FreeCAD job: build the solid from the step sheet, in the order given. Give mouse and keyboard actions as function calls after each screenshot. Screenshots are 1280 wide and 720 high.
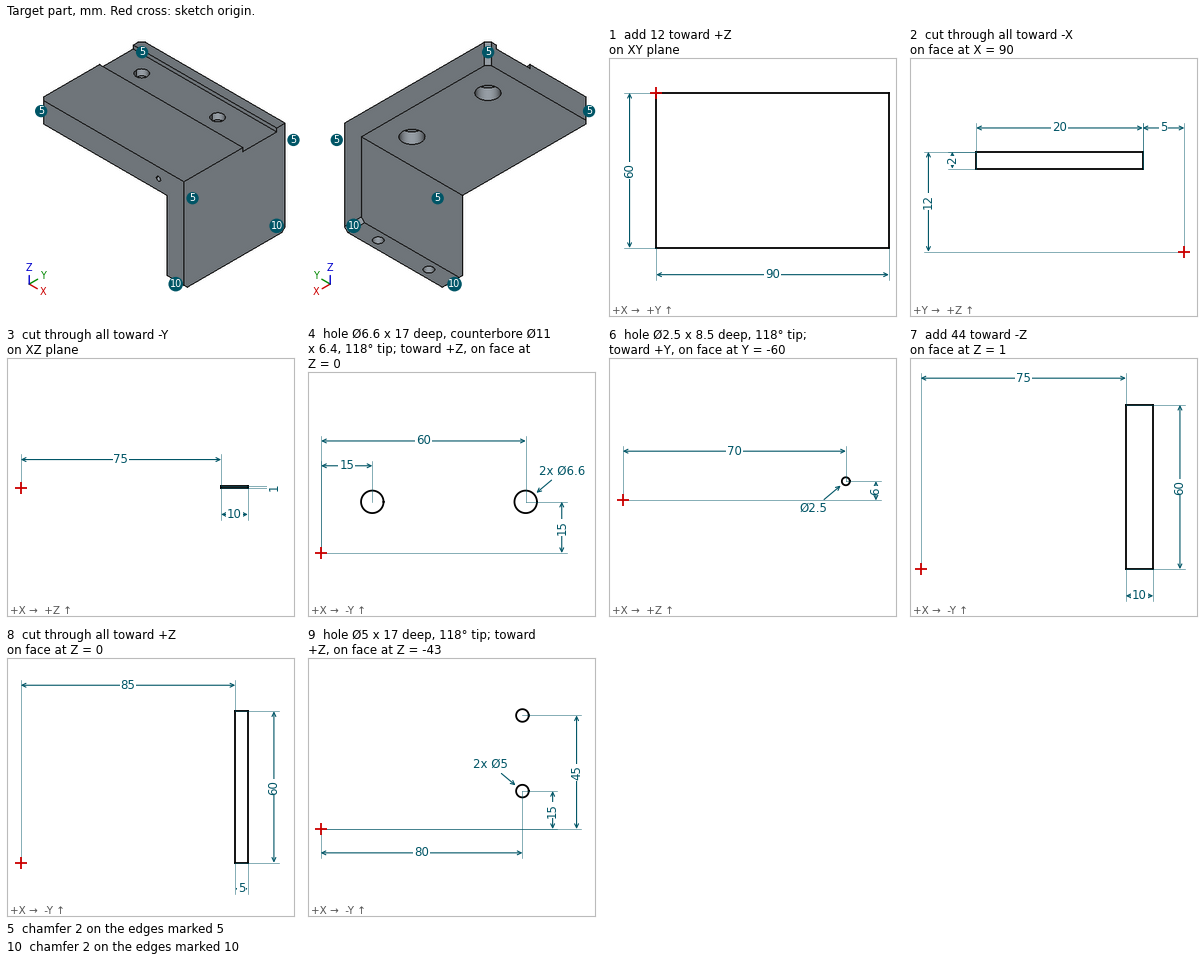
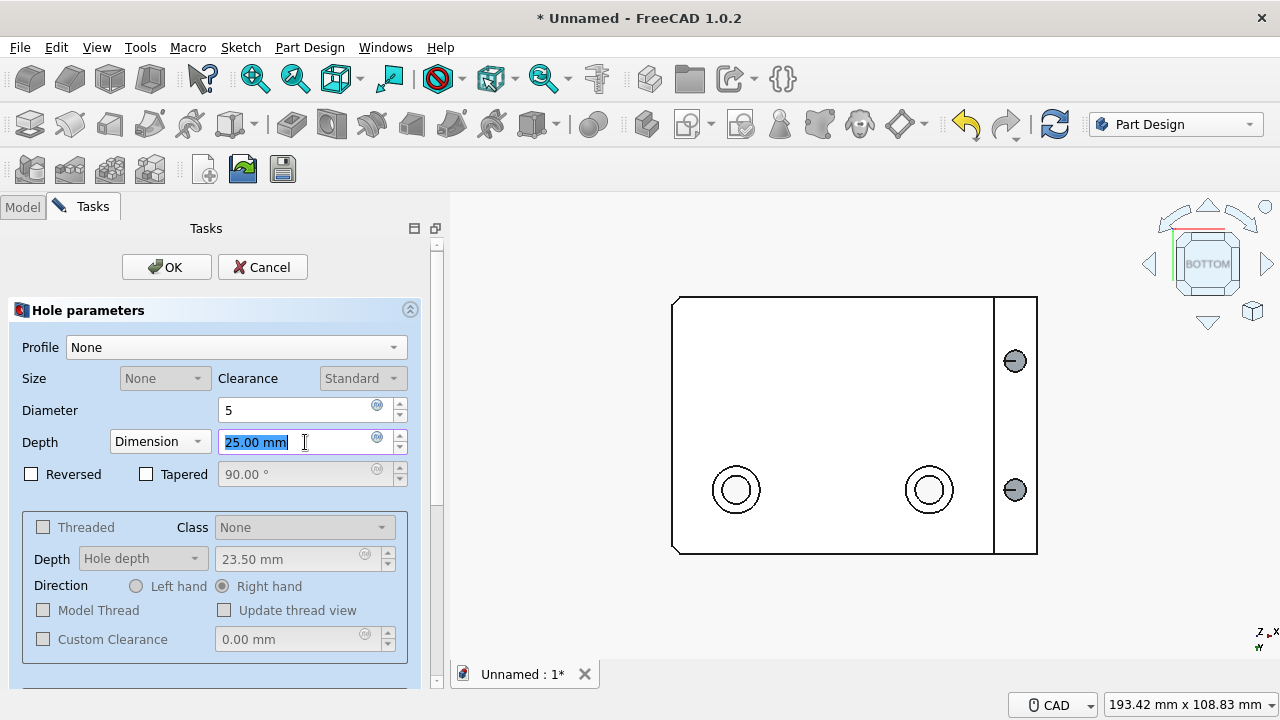
text(17)
key(Tab)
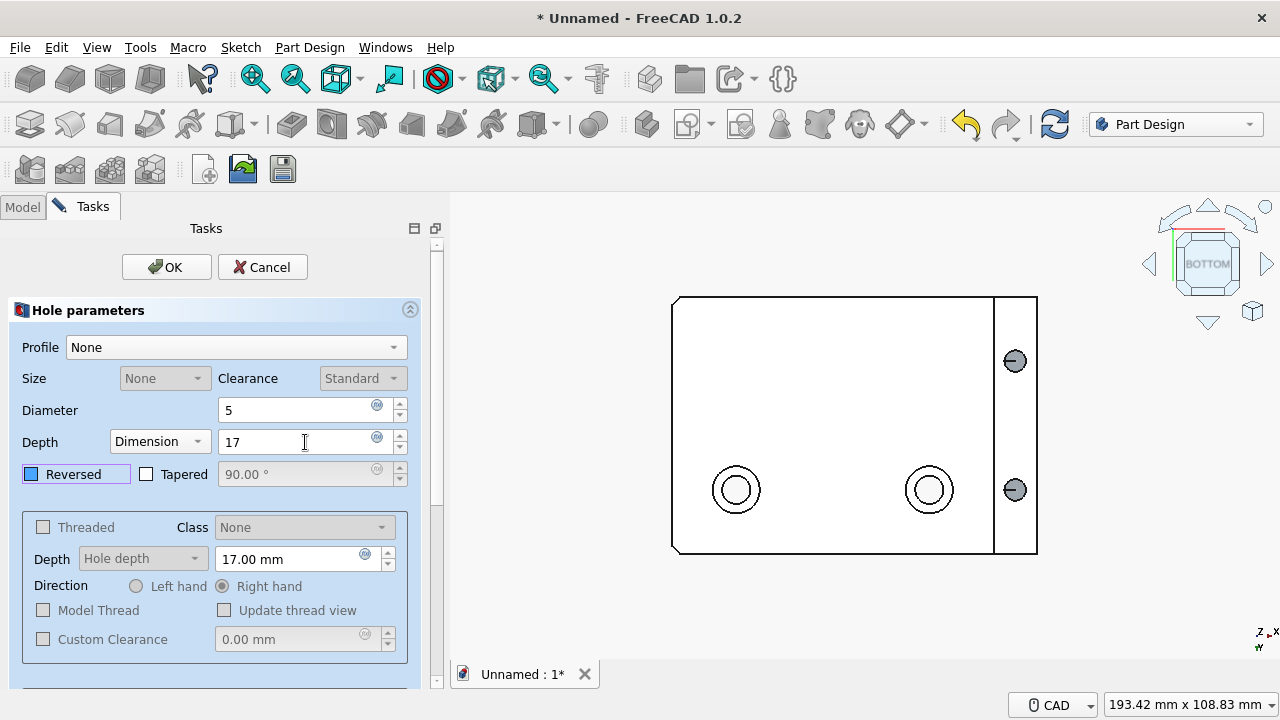
click(167, 267)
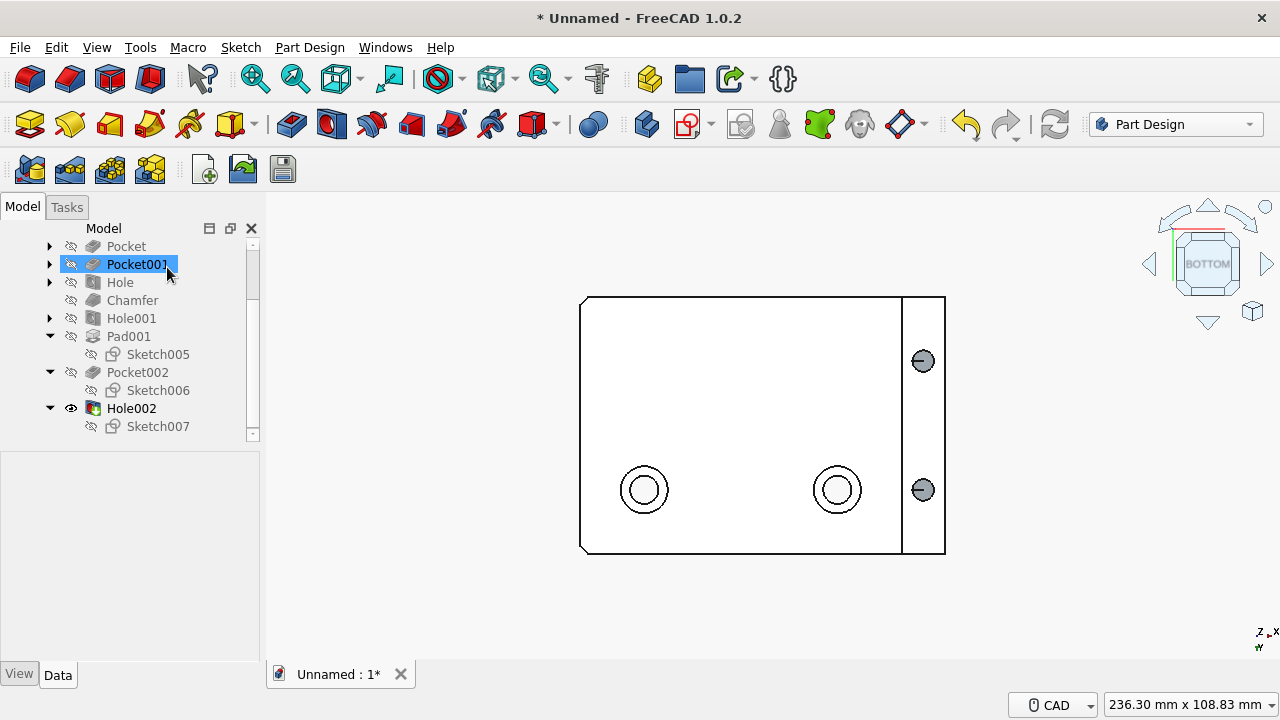
click(923, 553)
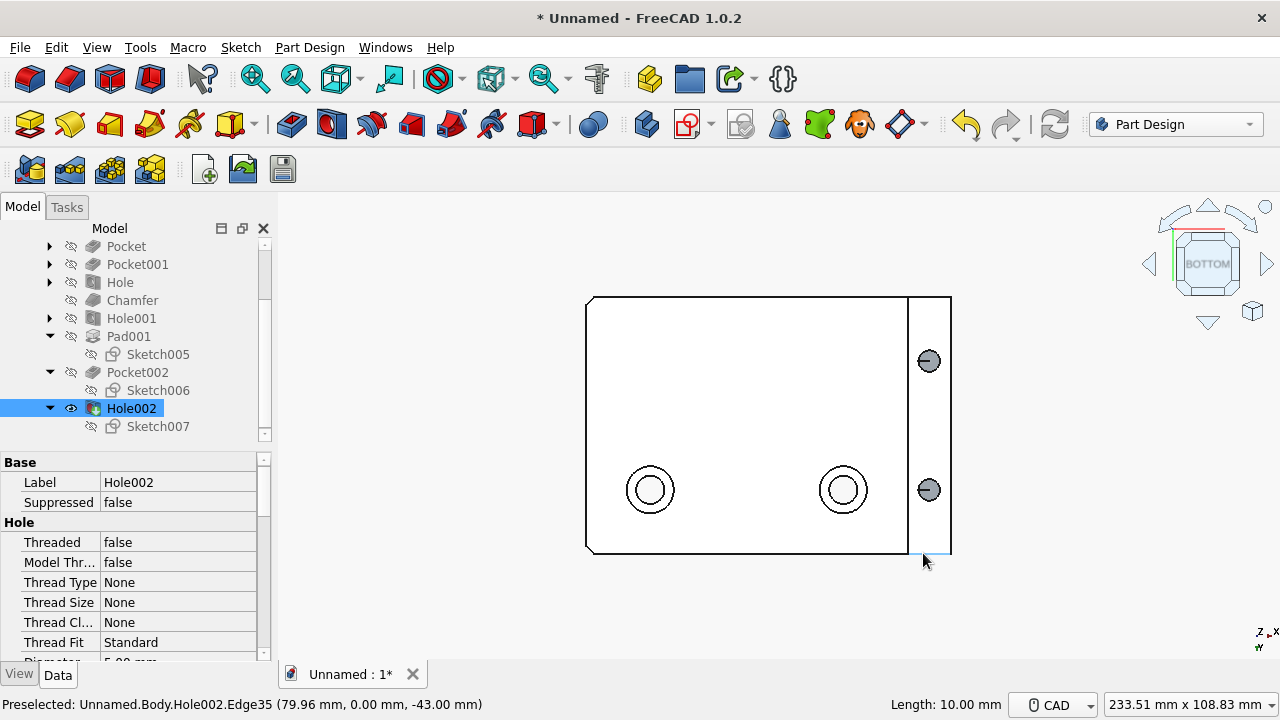
key(0)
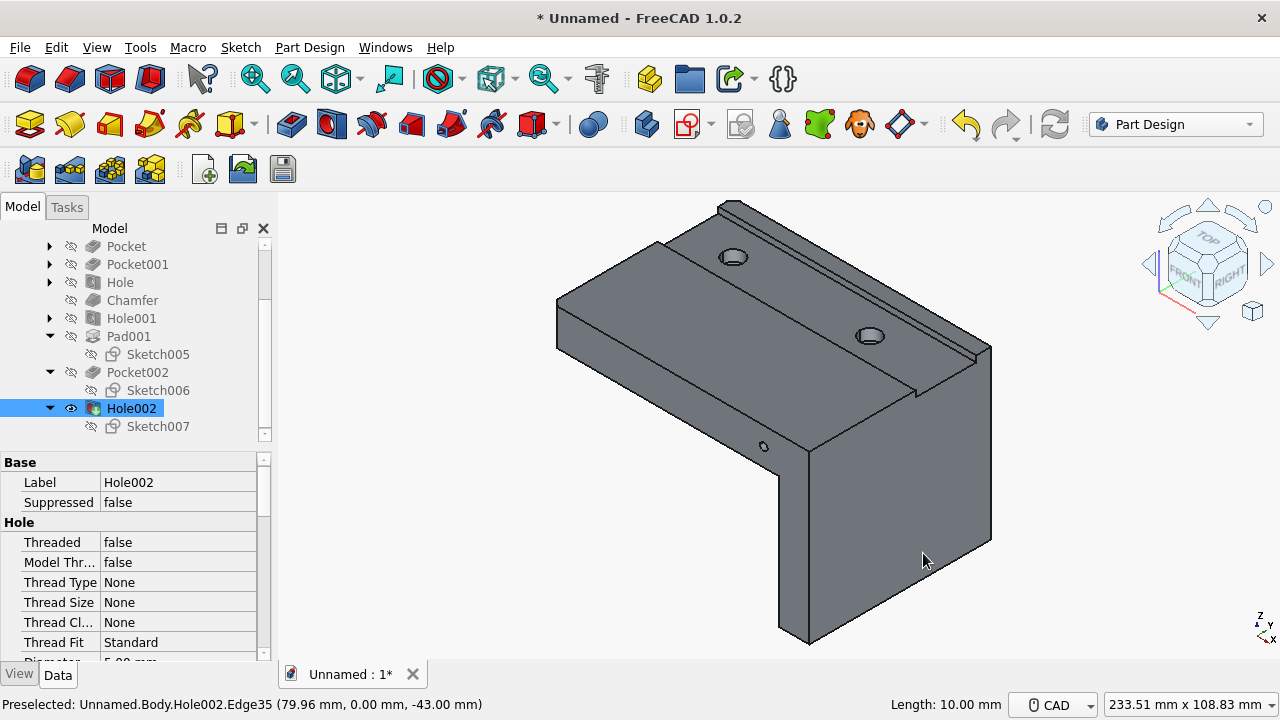
key(2)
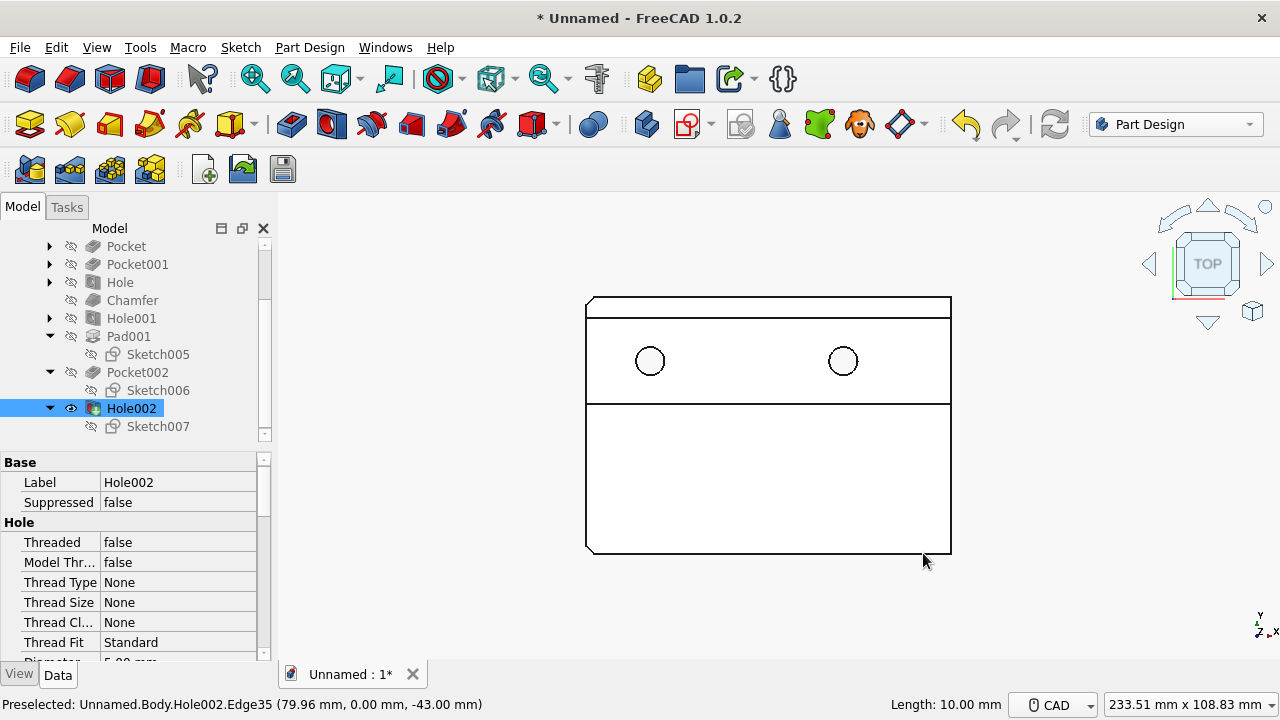
key(1)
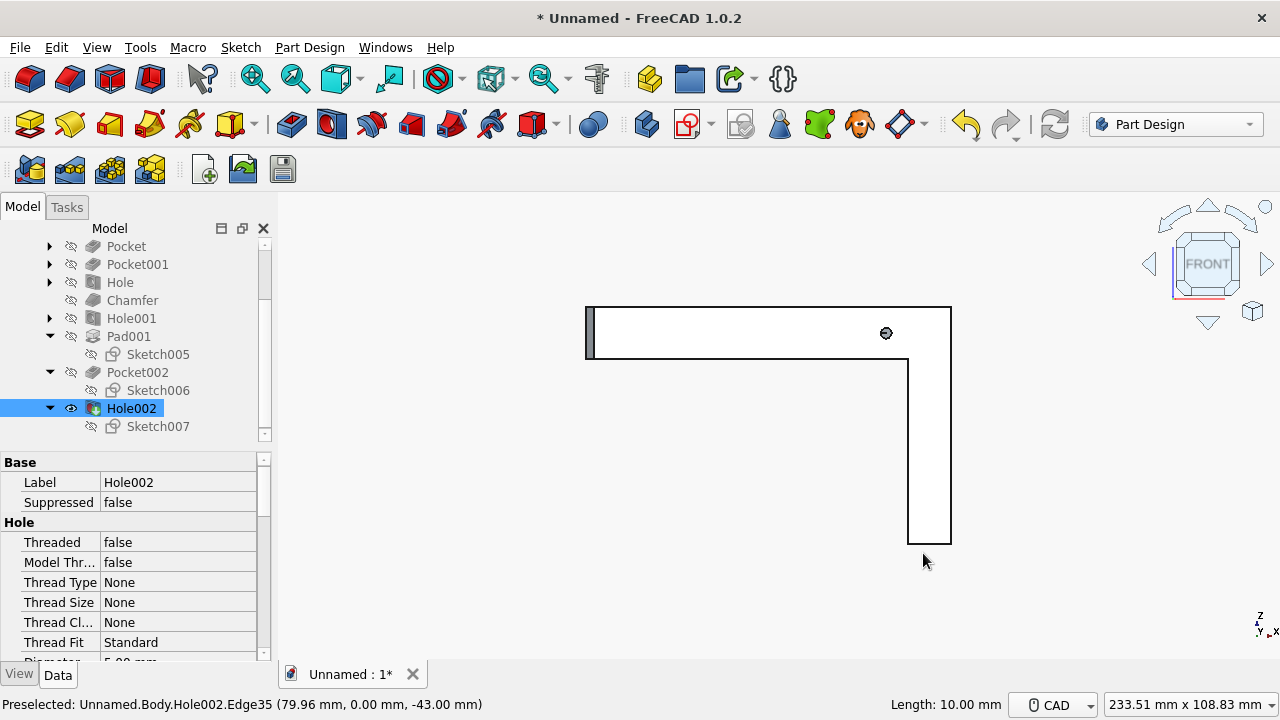
click(929, 543, ctrl)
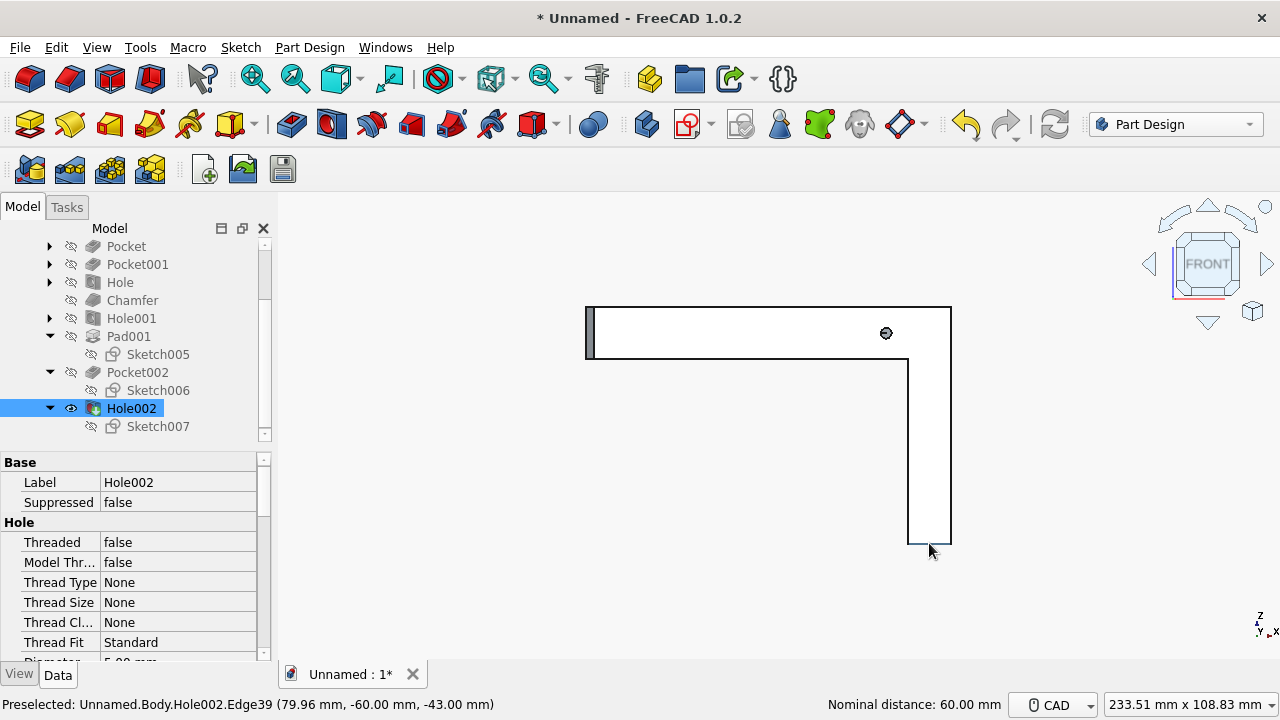
click(70, 80)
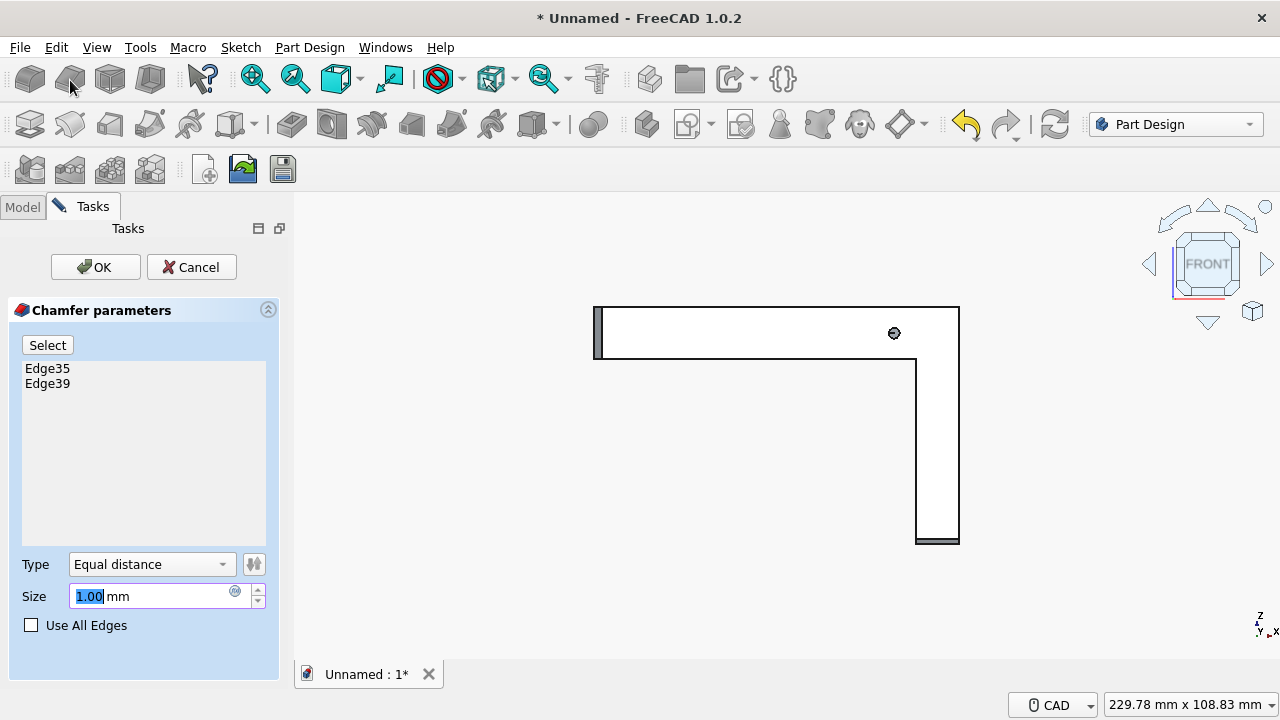
text(2)
key(Tab)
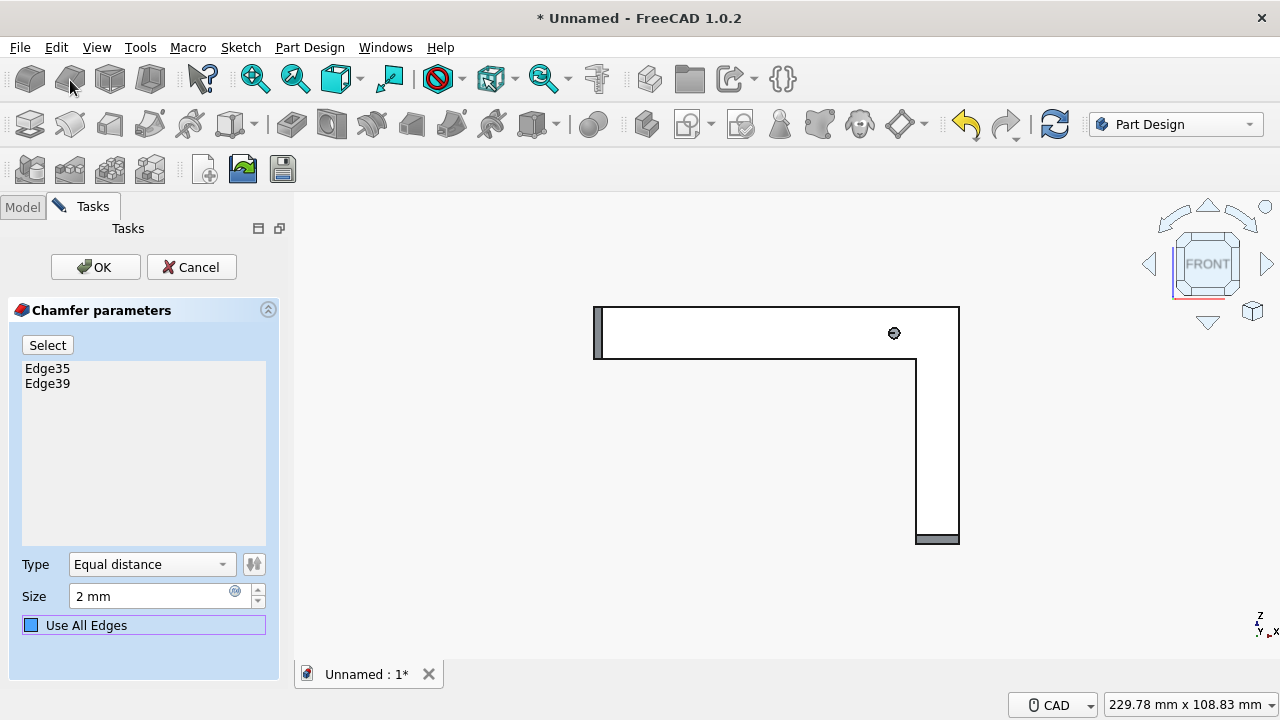
click(96, 267)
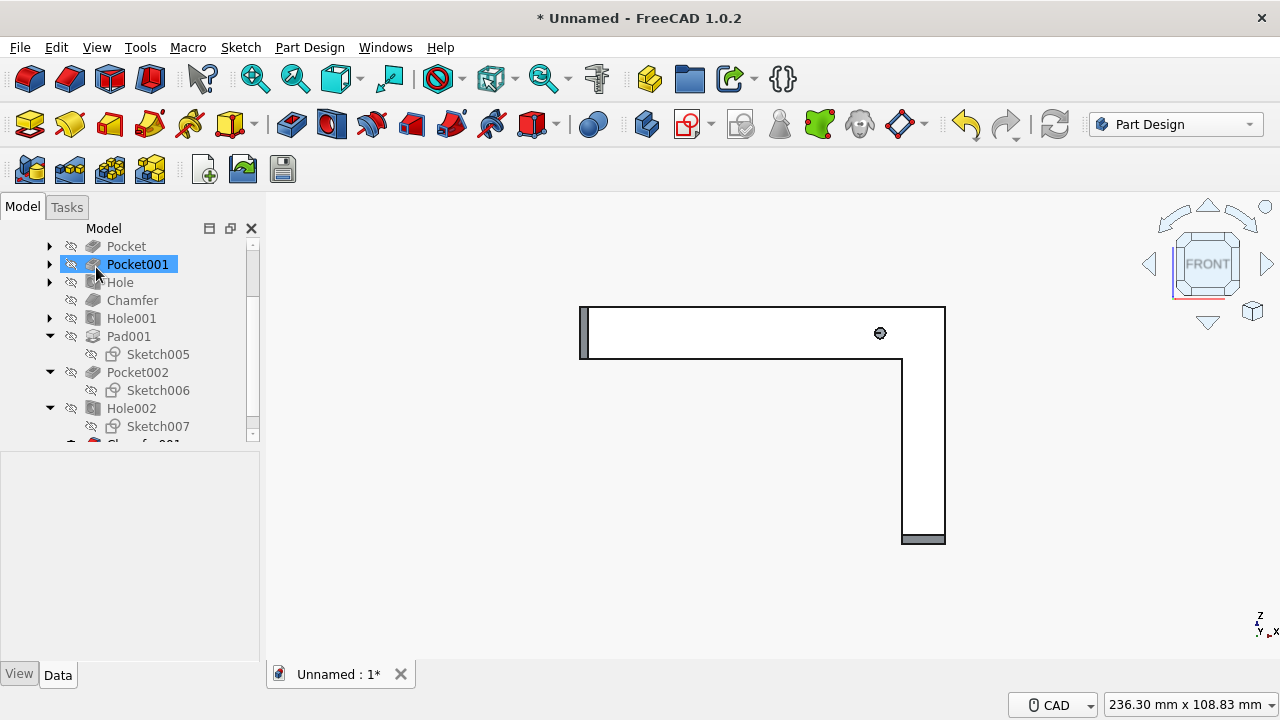
key(0)